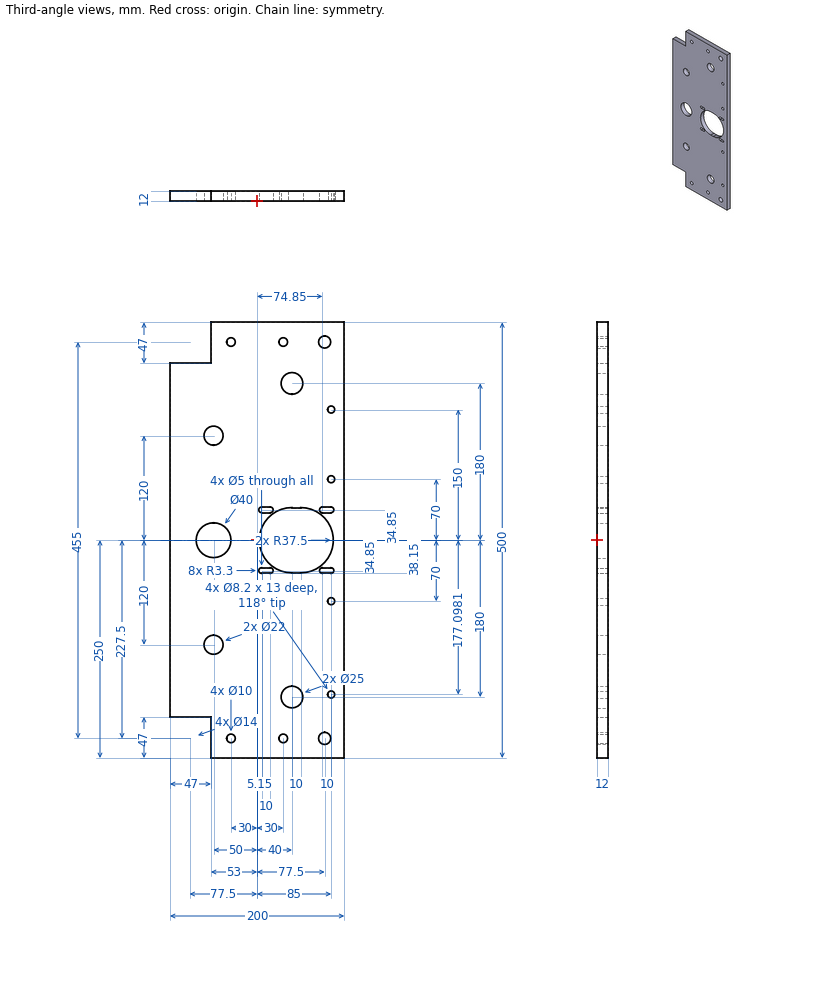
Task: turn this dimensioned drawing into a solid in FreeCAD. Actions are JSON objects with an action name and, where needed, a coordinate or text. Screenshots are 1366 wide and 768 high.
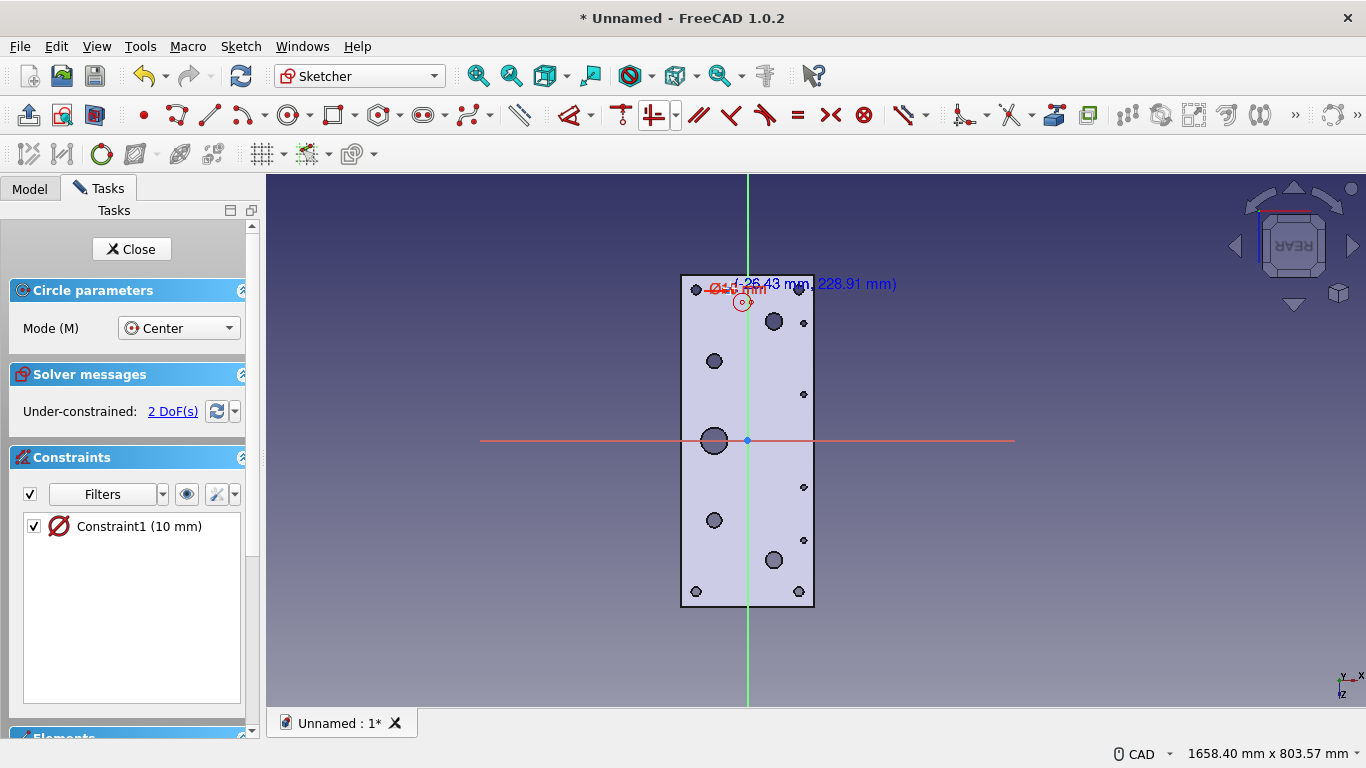
{"action": "scroll", "coordinate": [767, 290], "scroll_direction": "up", "scroll_amount": 10}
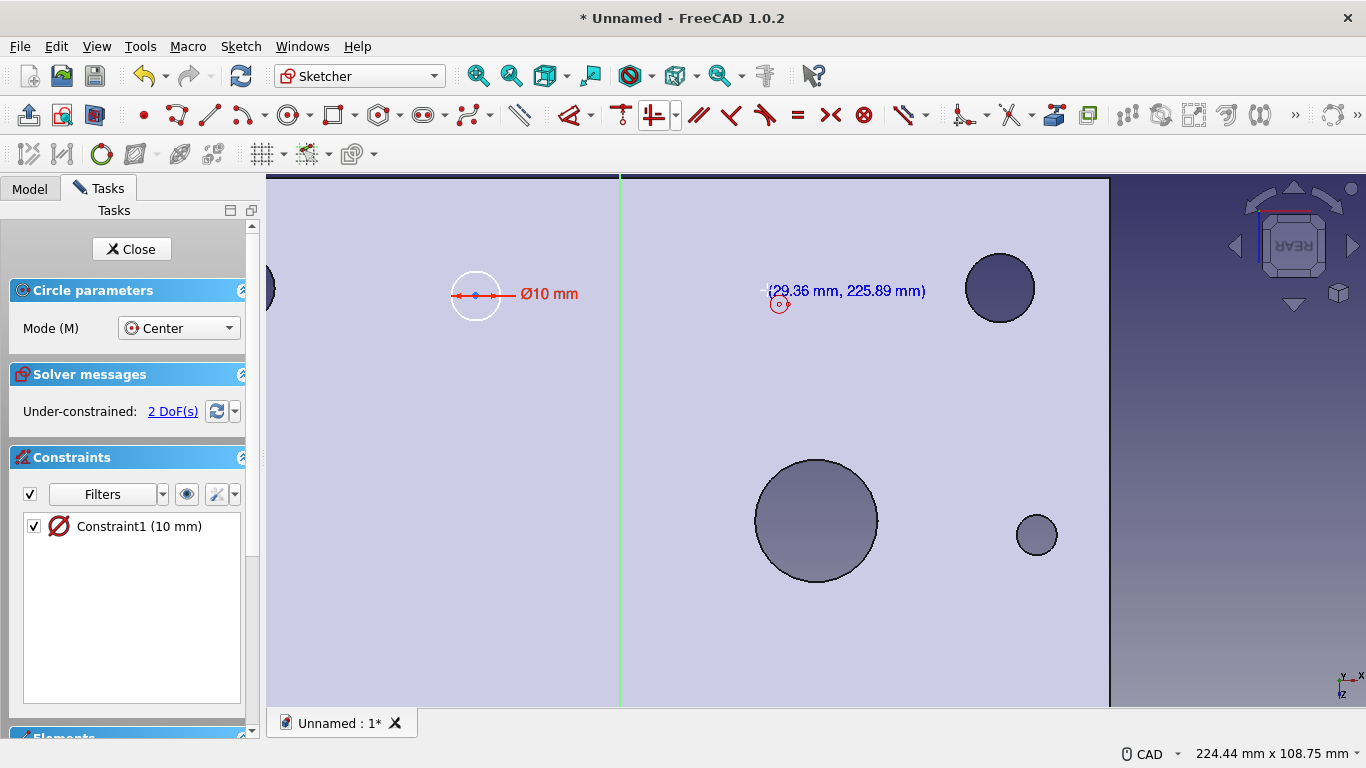
{"action": "scroll", "coordinate": [767, 290], "scroll_direction": "down", "scroll_amount": 10}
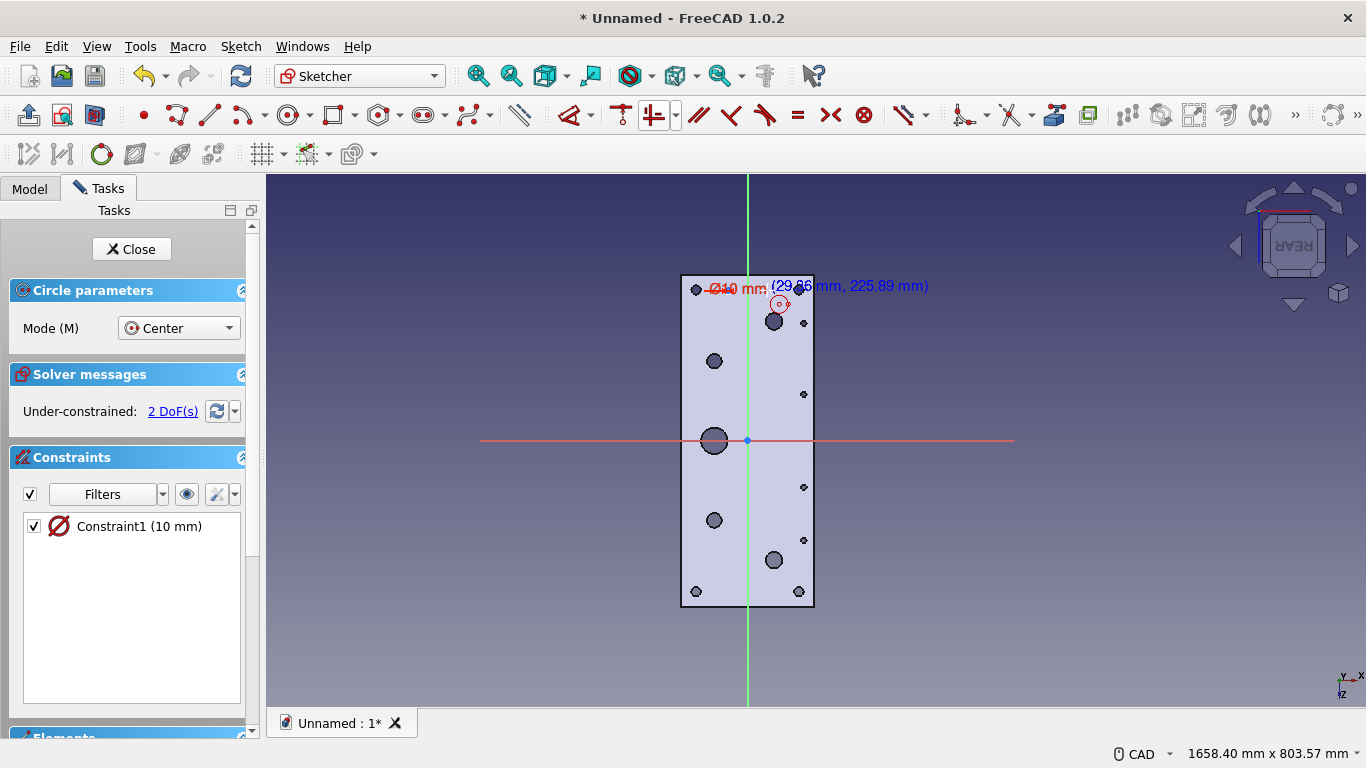
{"action": "left_click", "coordinate": [767, 290]}
{"action": "mouse_move", "coordinate": [770, 288]}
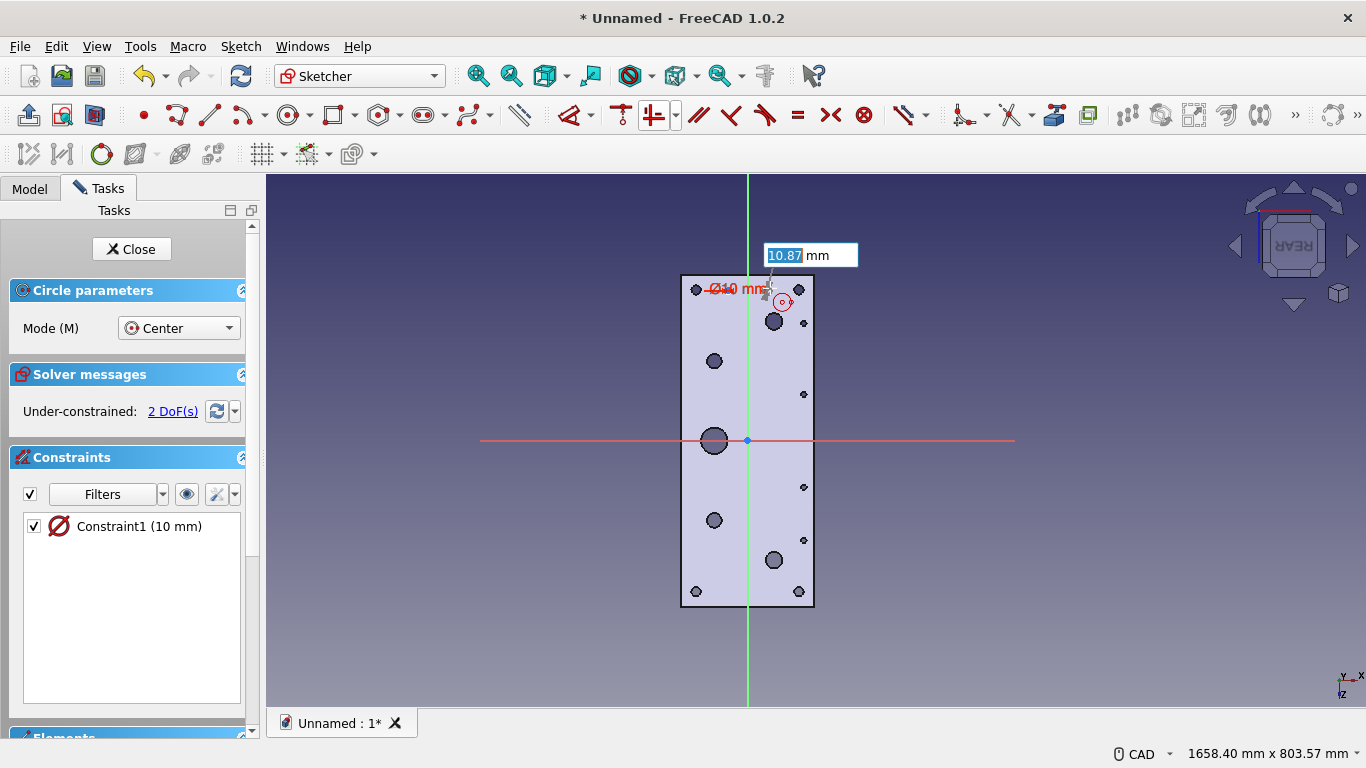
{"action": "type", "text": "10"}
{"action": "key", "text": "Return"}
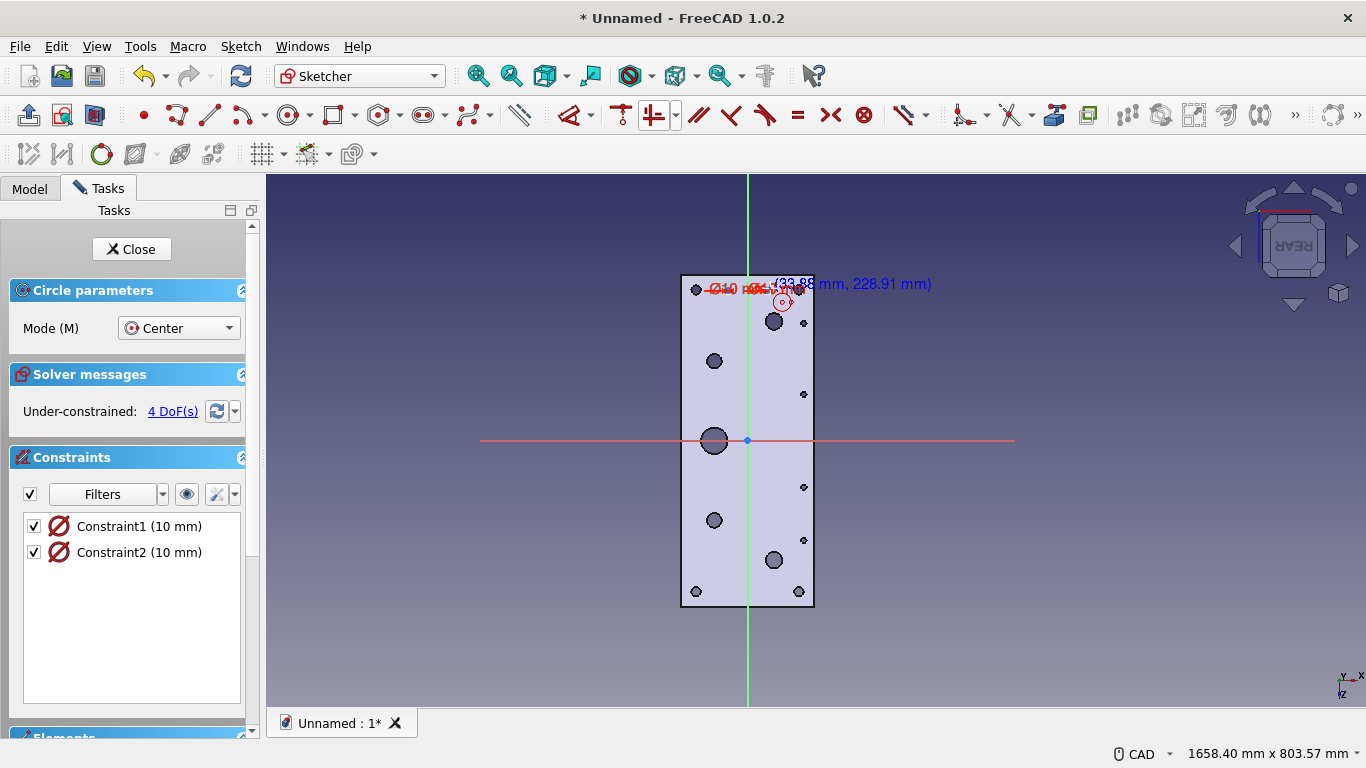
{"action": "scroll", "coordinate": [767, 592], "scroll_direction": "up", "scroll_amount": 10}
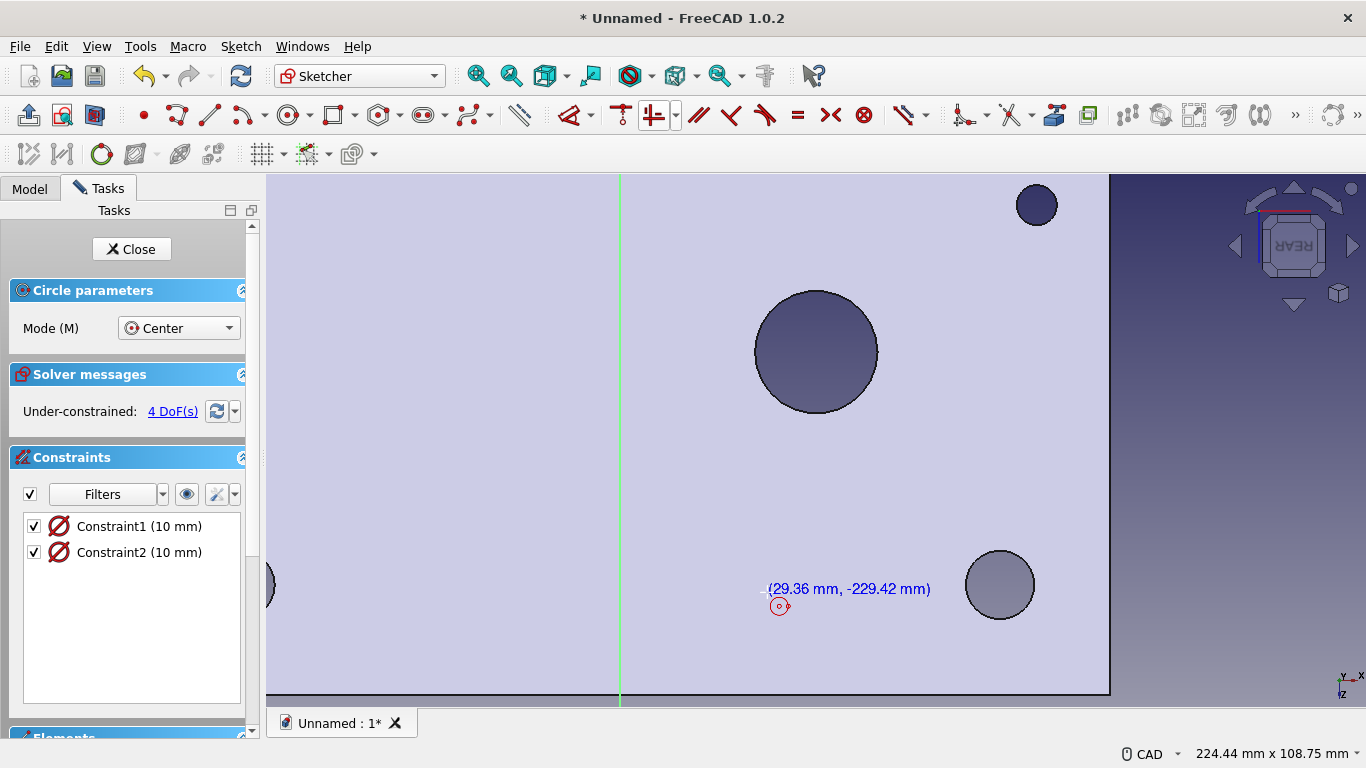
{"action": "scroll", "coordinate": [767, 592], "scroll_direction": "down", "scroll_amount": 10}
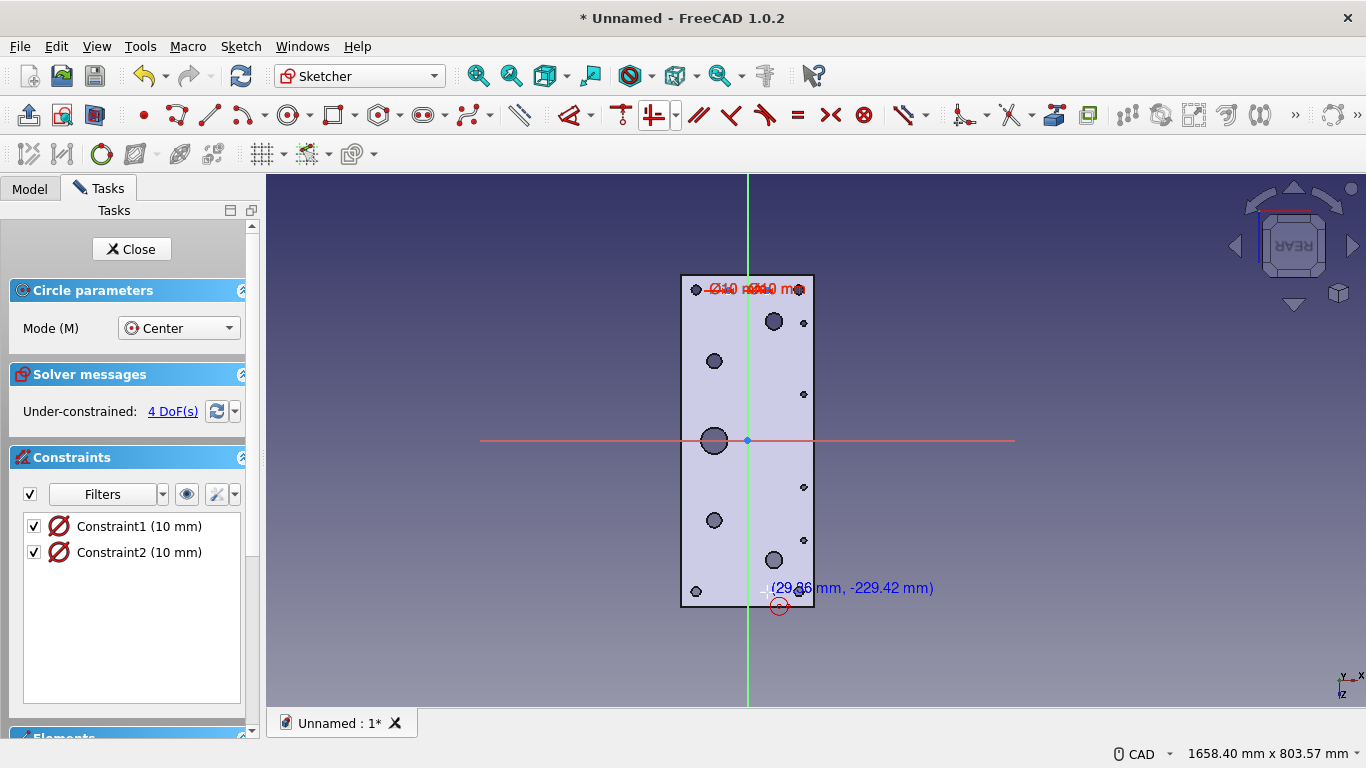
{"action": "left_click", "coordinate": [767, 592]}
{"action": "mouse_move", "coordinate": [770, 589]}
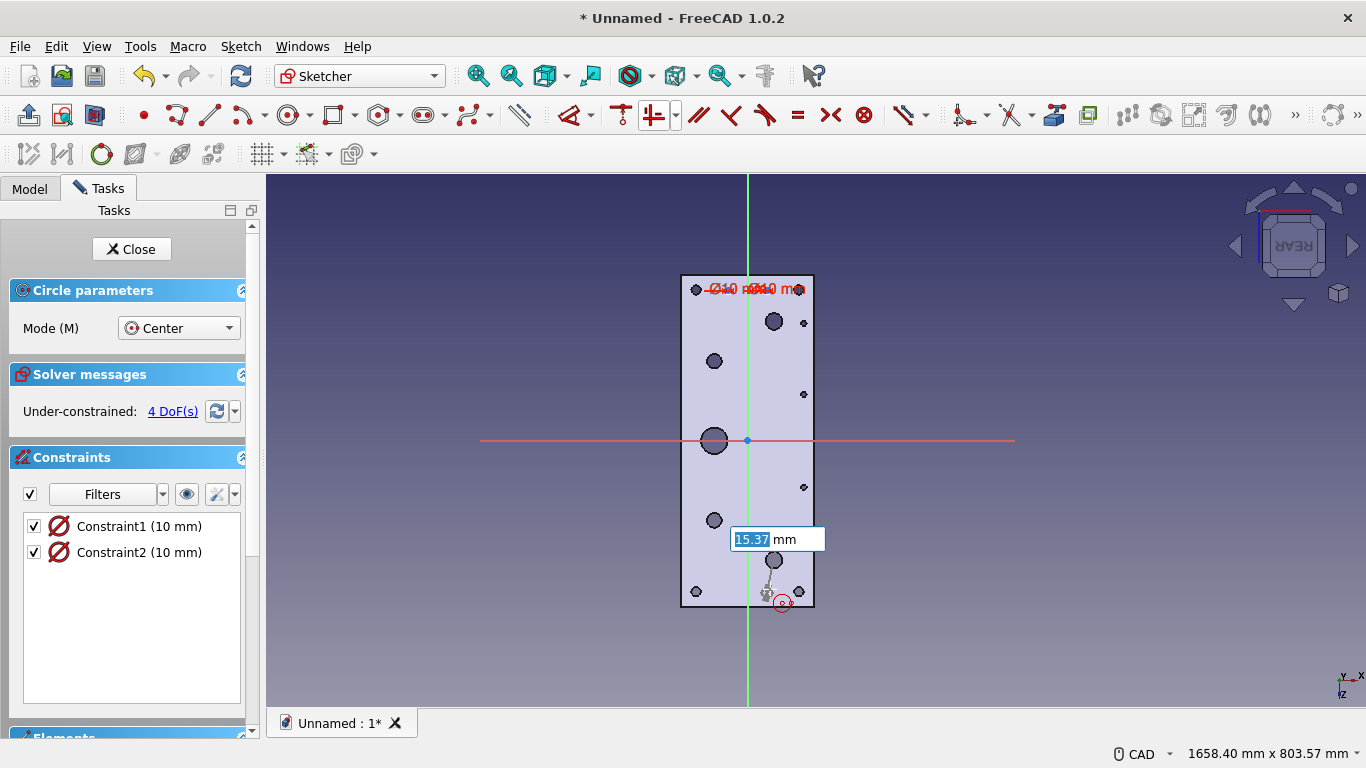
{"action": "type", "text": "10"}
{"action": "key", "text": "Return"}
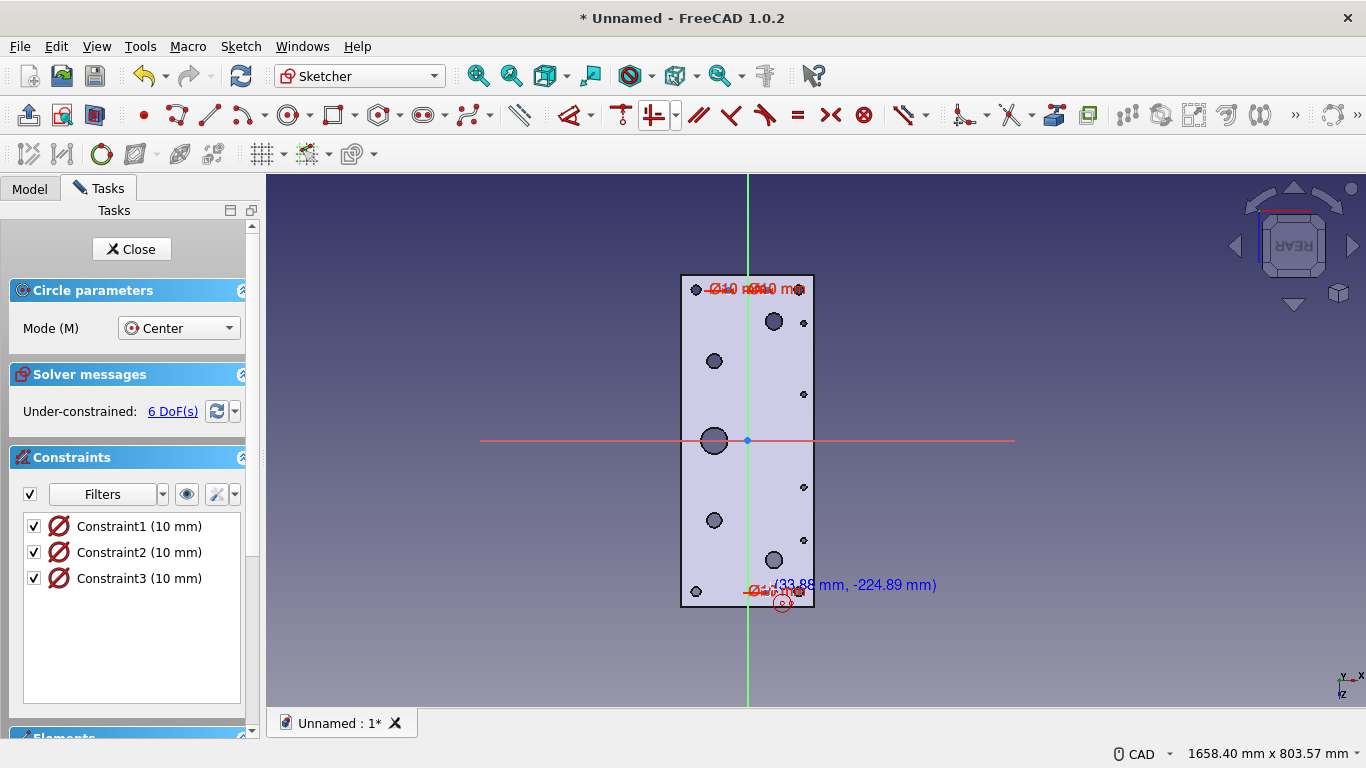
{"action": "scroll", "coordinate": [728, 592], "scroll_direction": "up", "scroll_amount": 10}